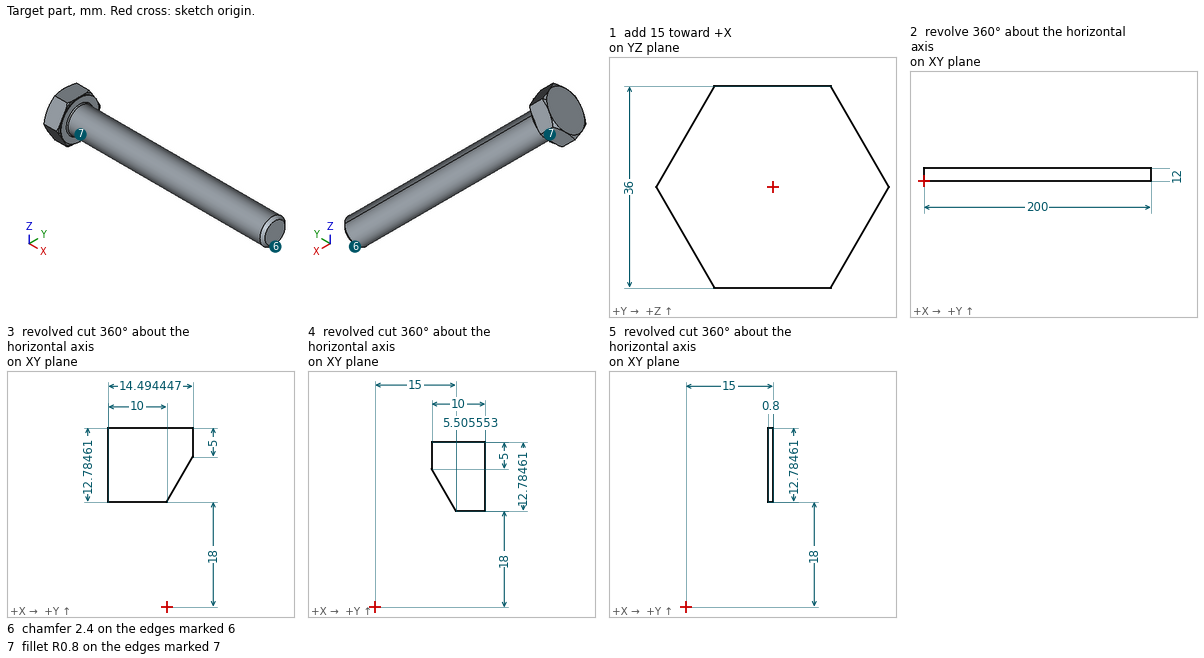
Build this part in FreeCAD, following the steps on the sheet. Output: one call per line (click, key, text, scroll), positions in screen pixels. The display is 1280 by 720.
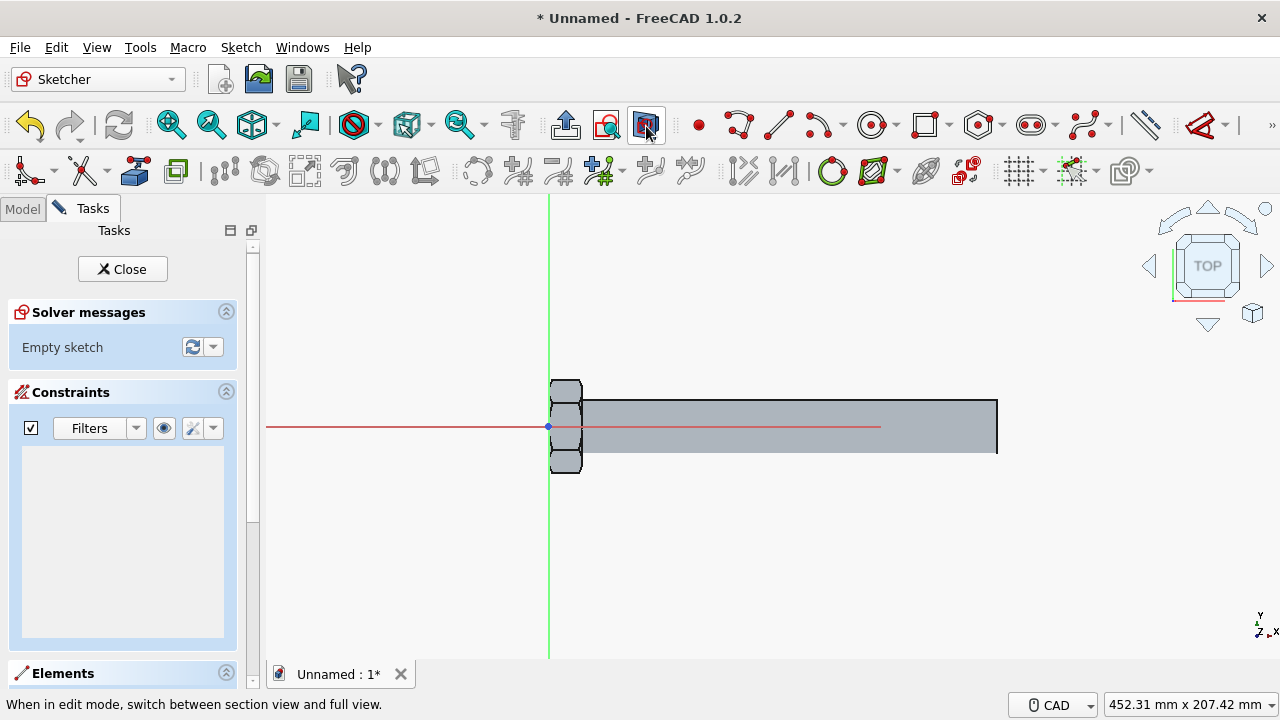
scroll(520, 381, up, 7)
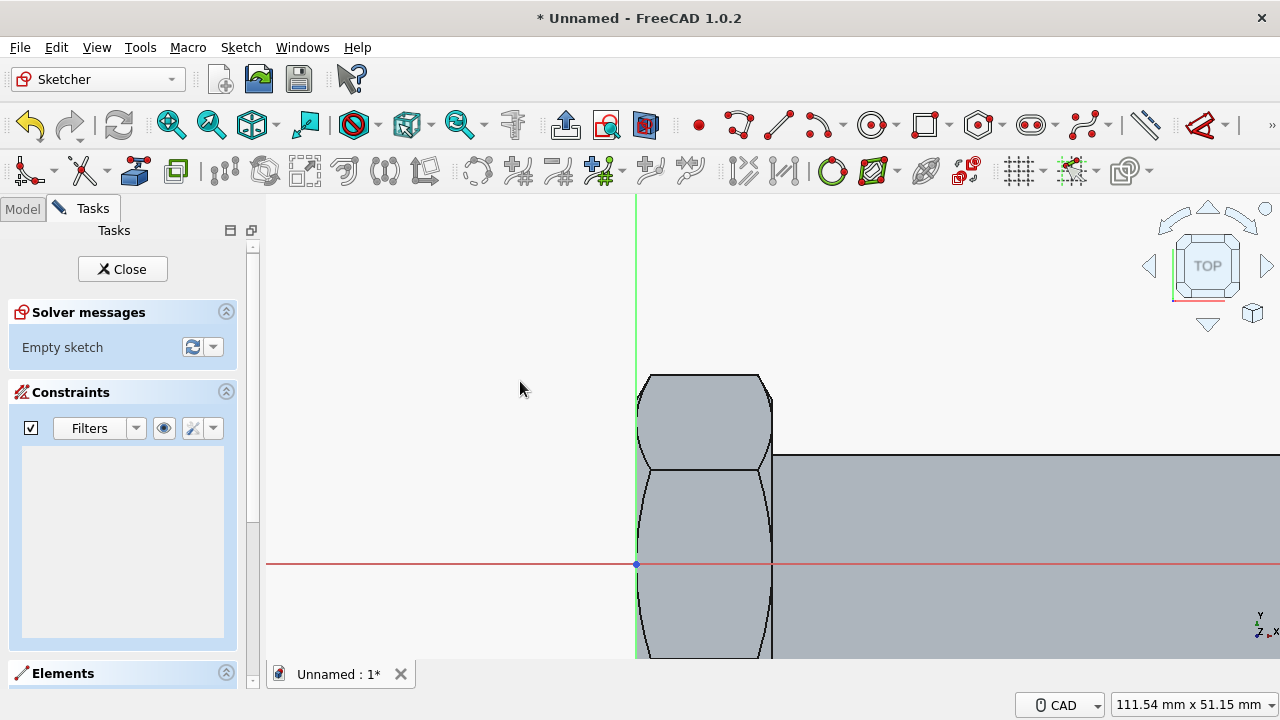
key(g)
key(r)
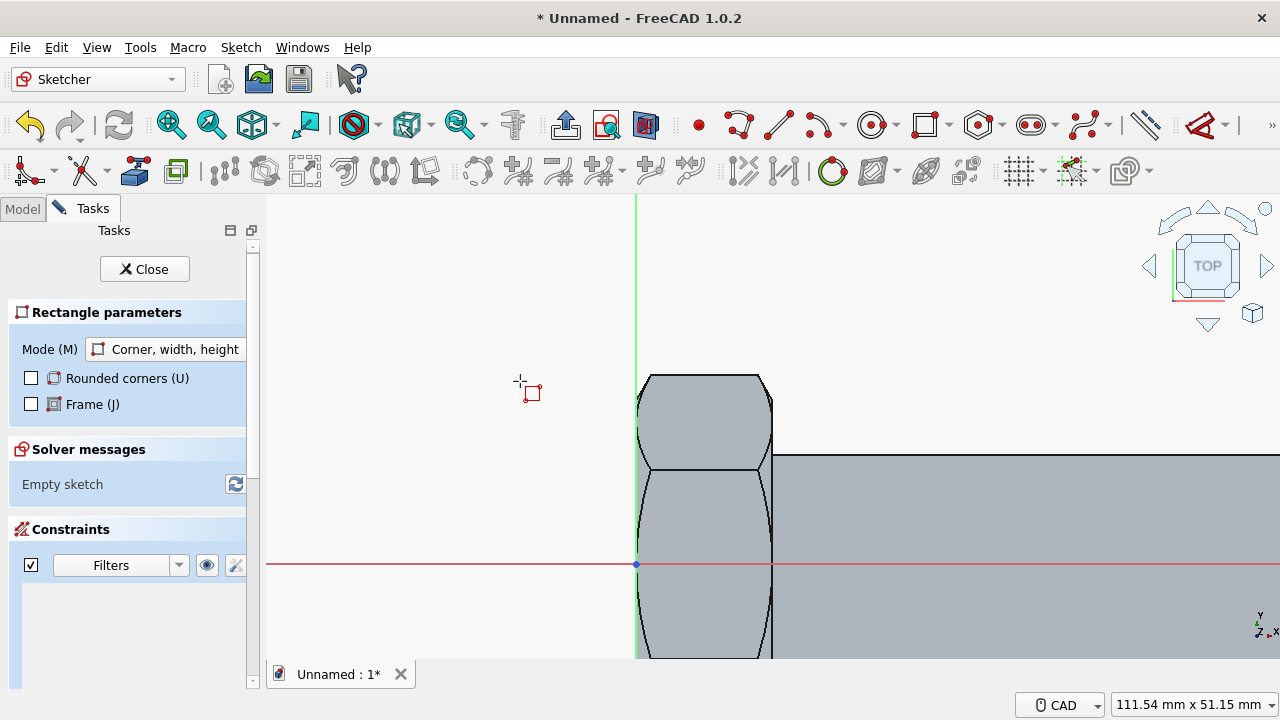
scroll(765, 284, up, 4)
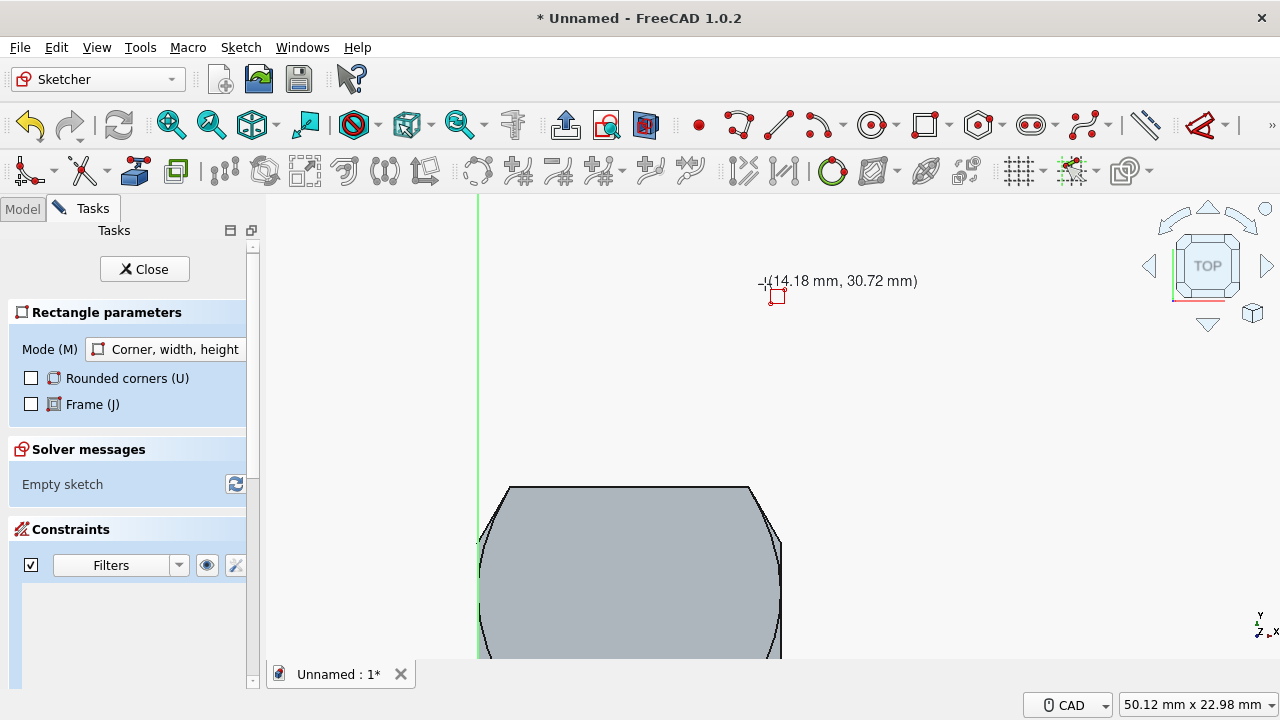
click(765, 285)
click(781, 543)
key(Escape)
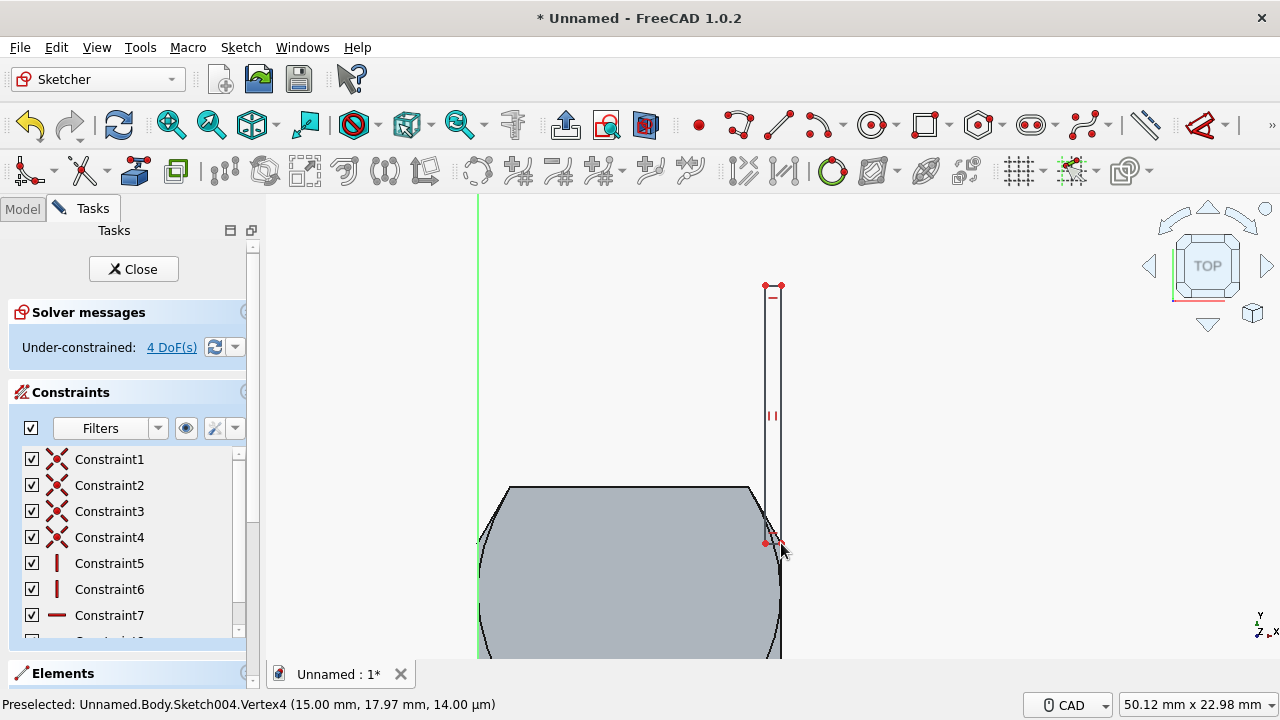
key(d)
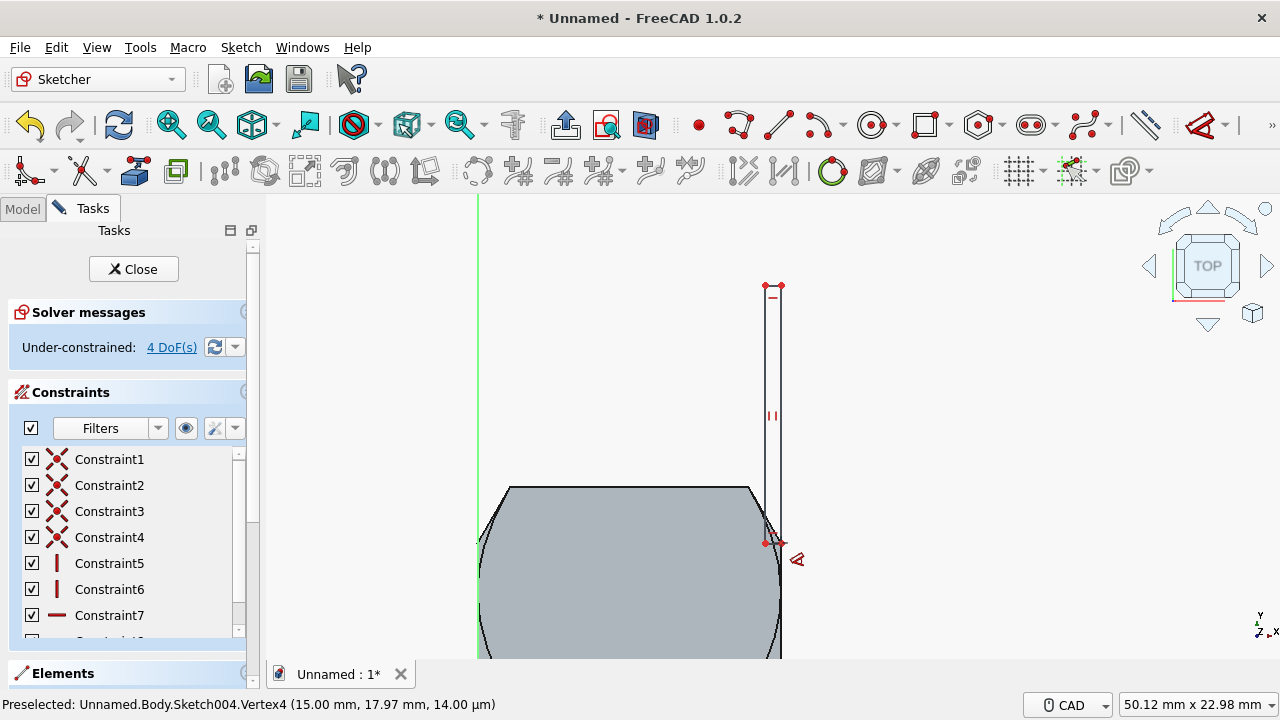
scroll(773, 544, up, 5)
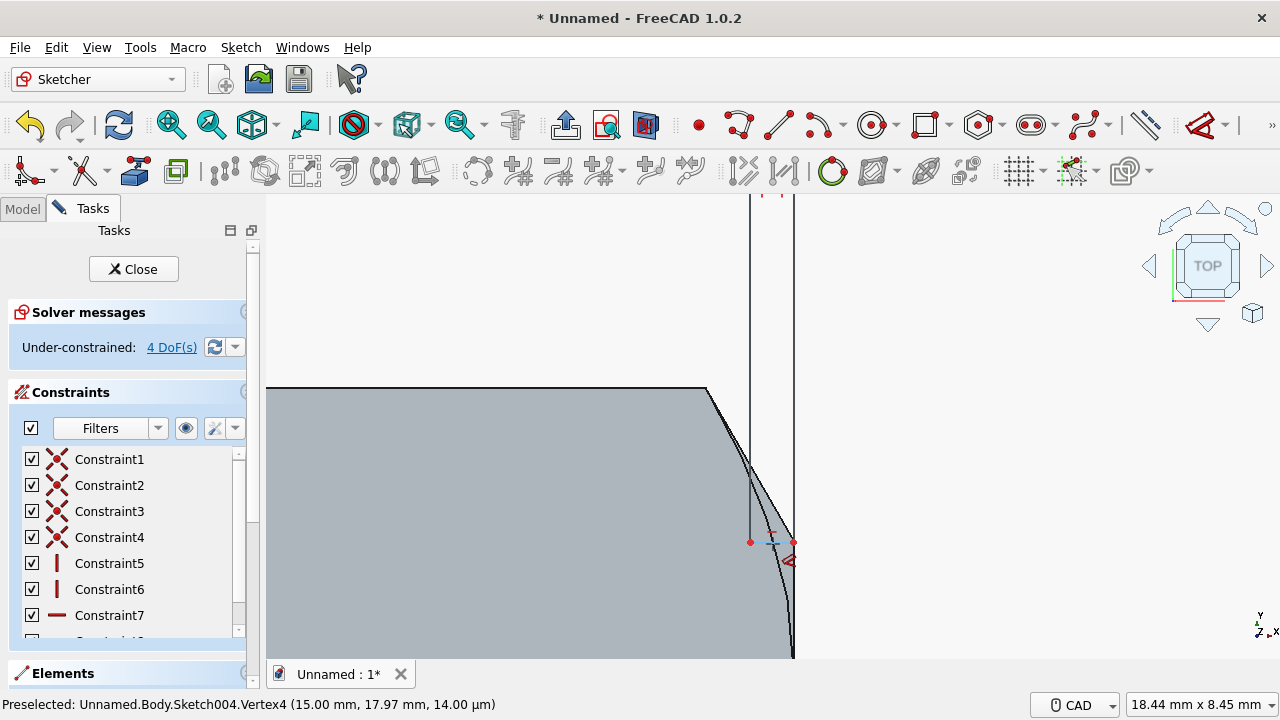
click(772, 543)
click(772, 509)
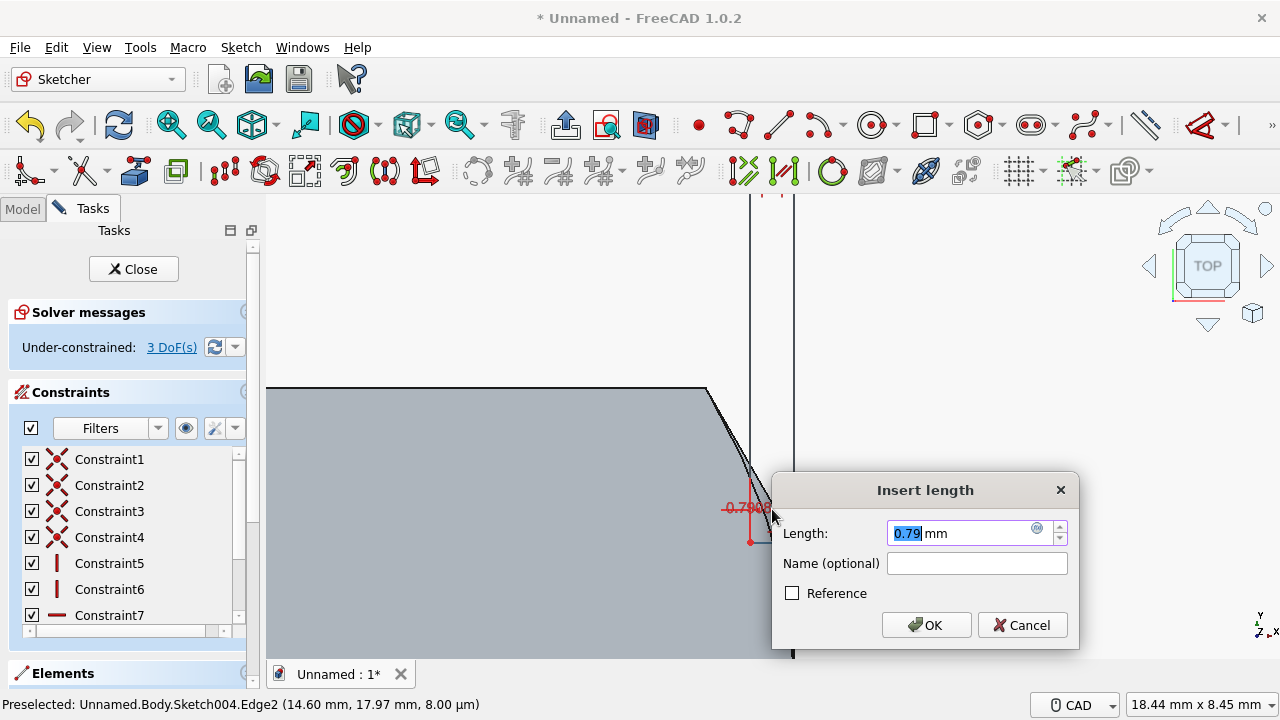
text(0.8)
key(Return)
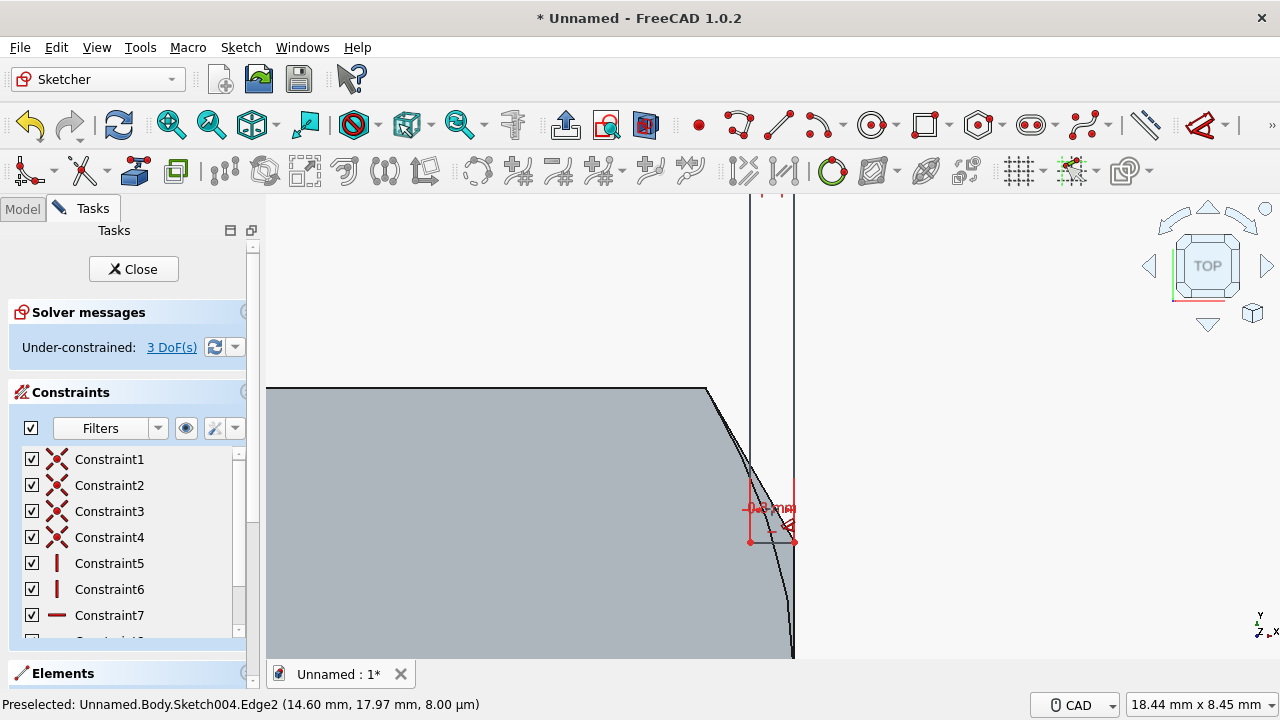
scroll(768, 375, down, 9)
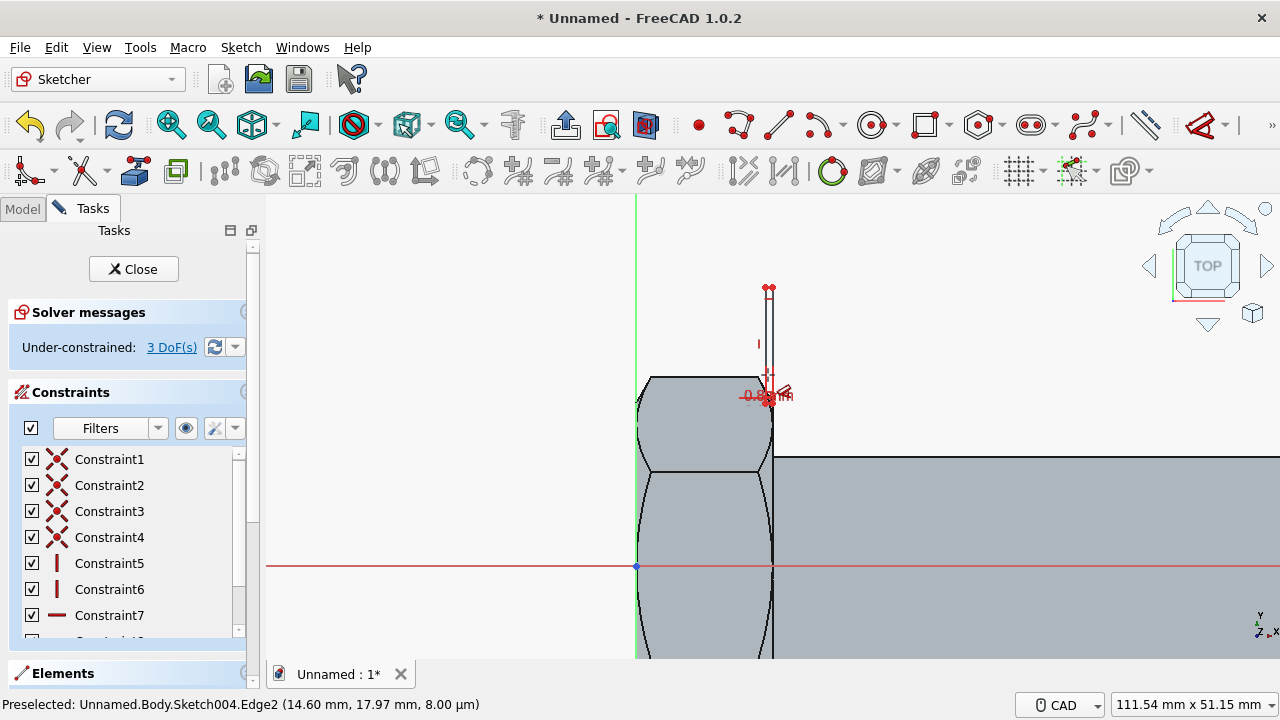
scroll(766, 403, up, 3)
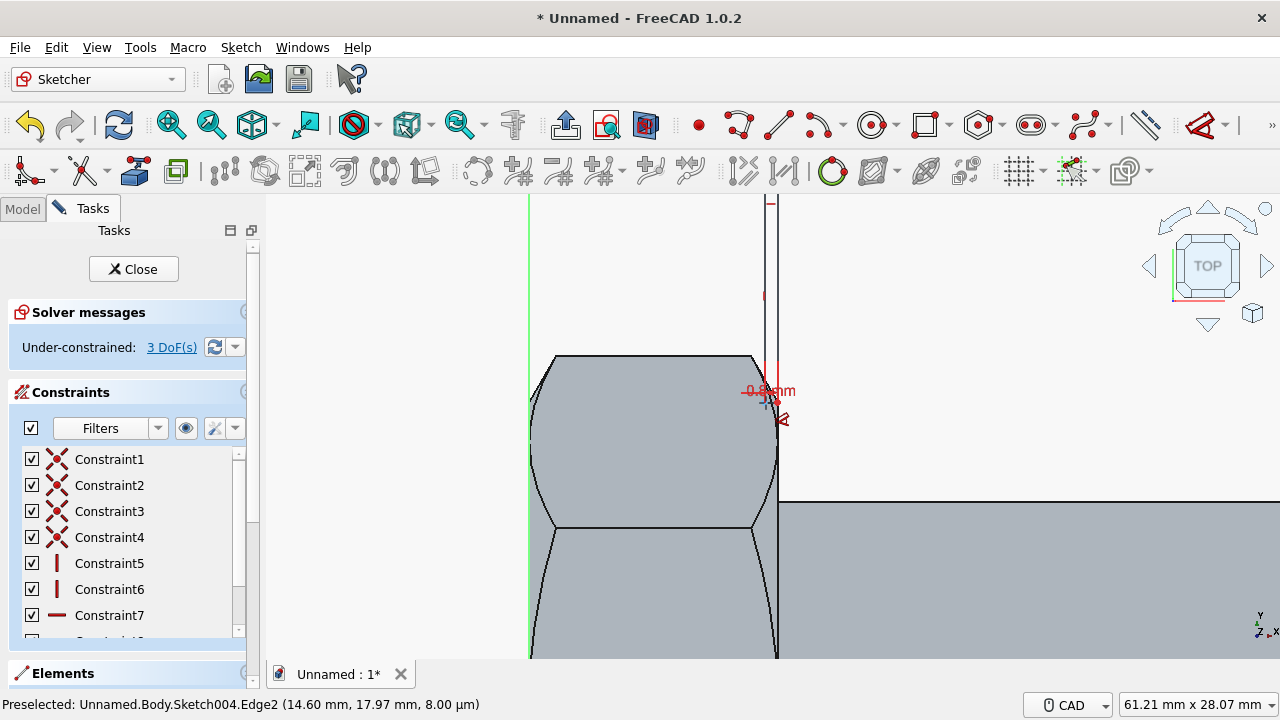
click(765, 403)
click(495, 517)